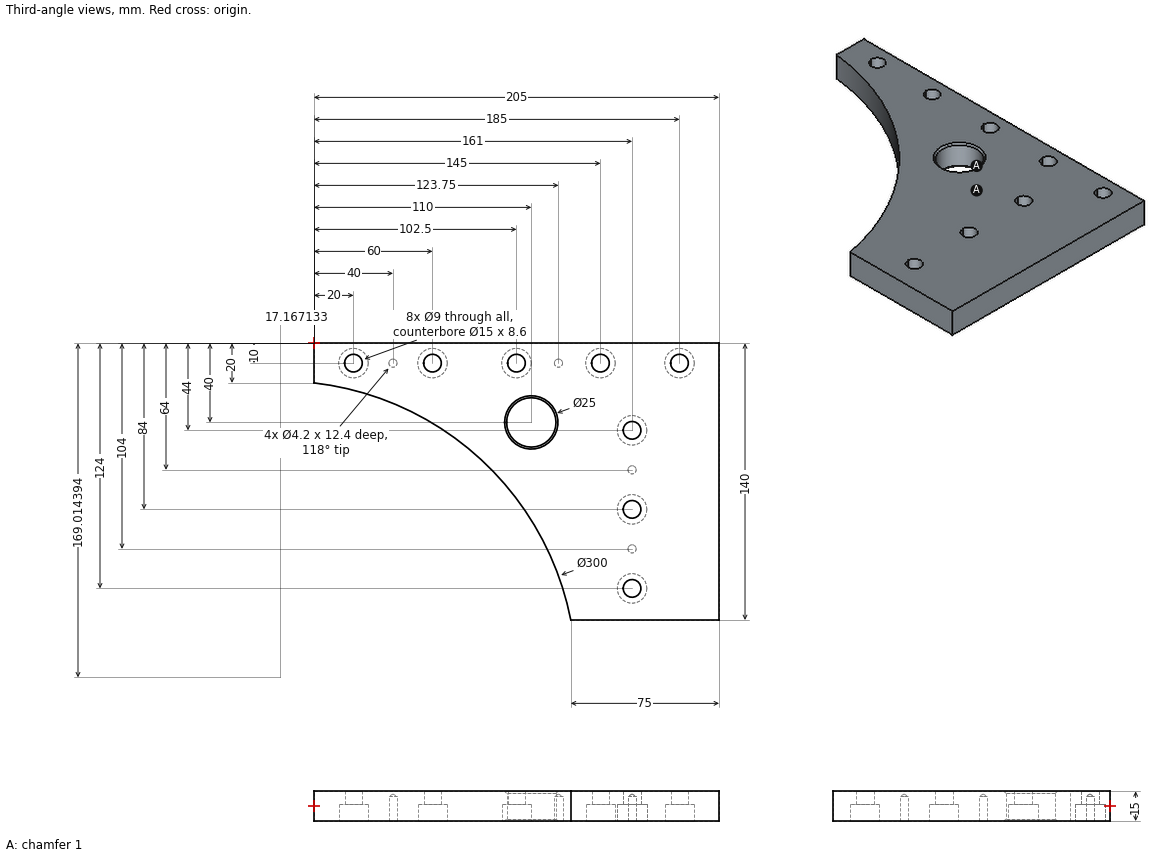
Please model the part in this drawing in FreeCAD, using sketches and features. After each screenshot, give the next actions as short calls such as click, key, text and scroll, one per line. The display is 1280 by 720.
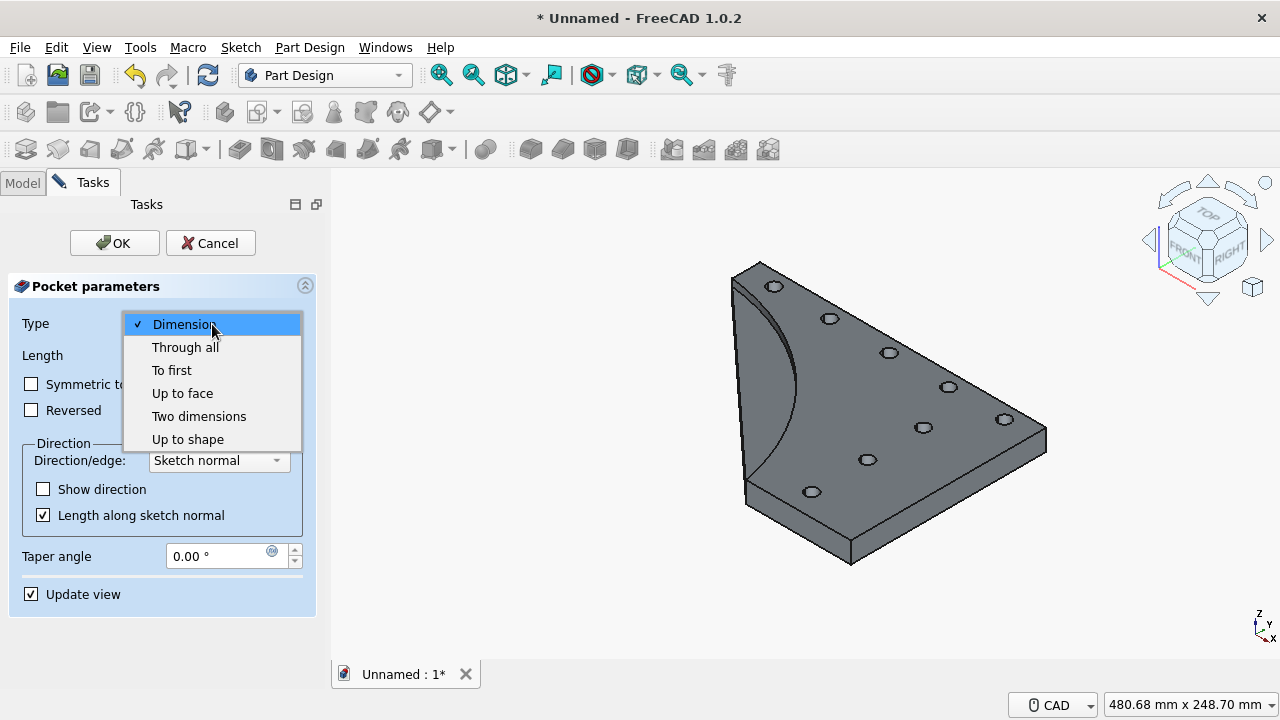
click(212, 348)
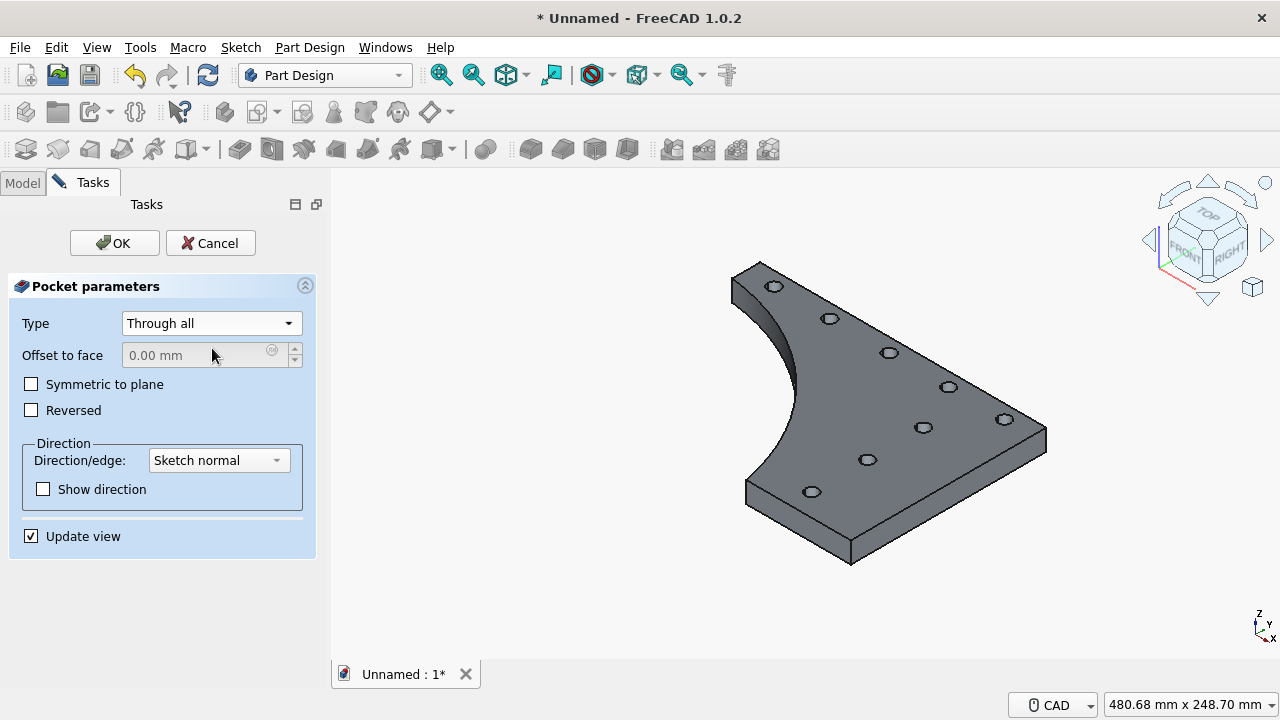
click(115, 243)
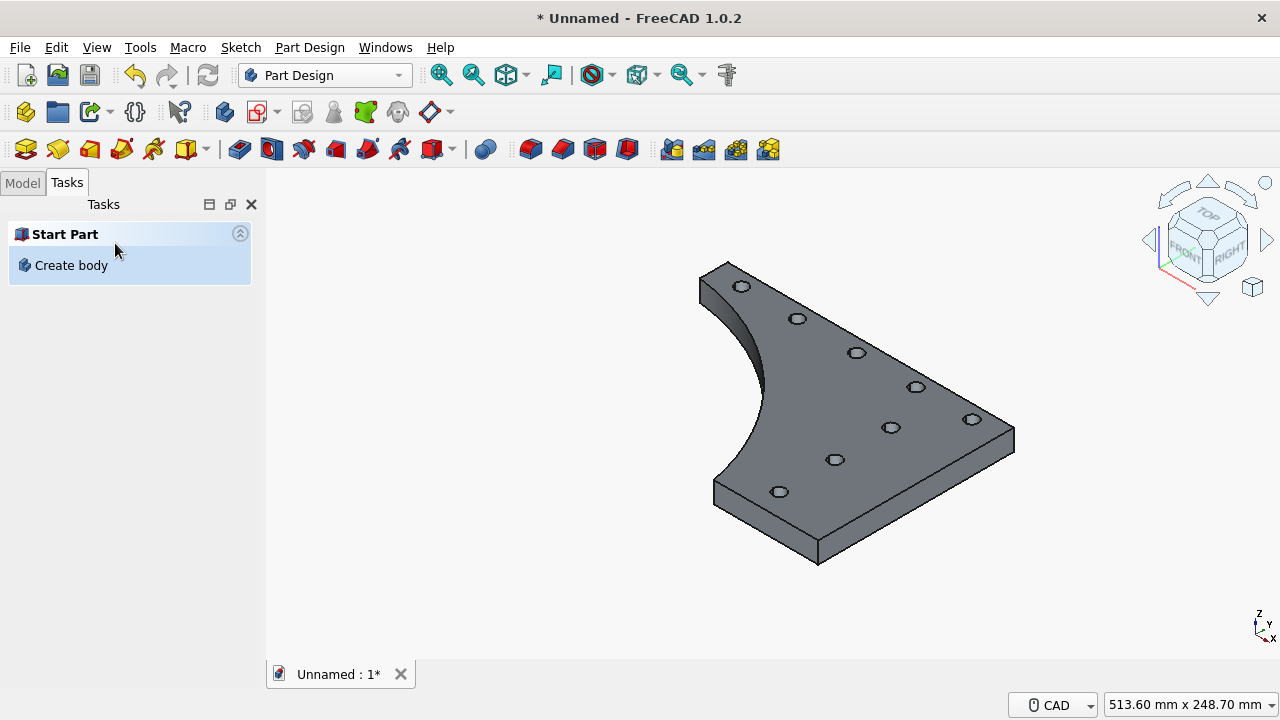
key(5)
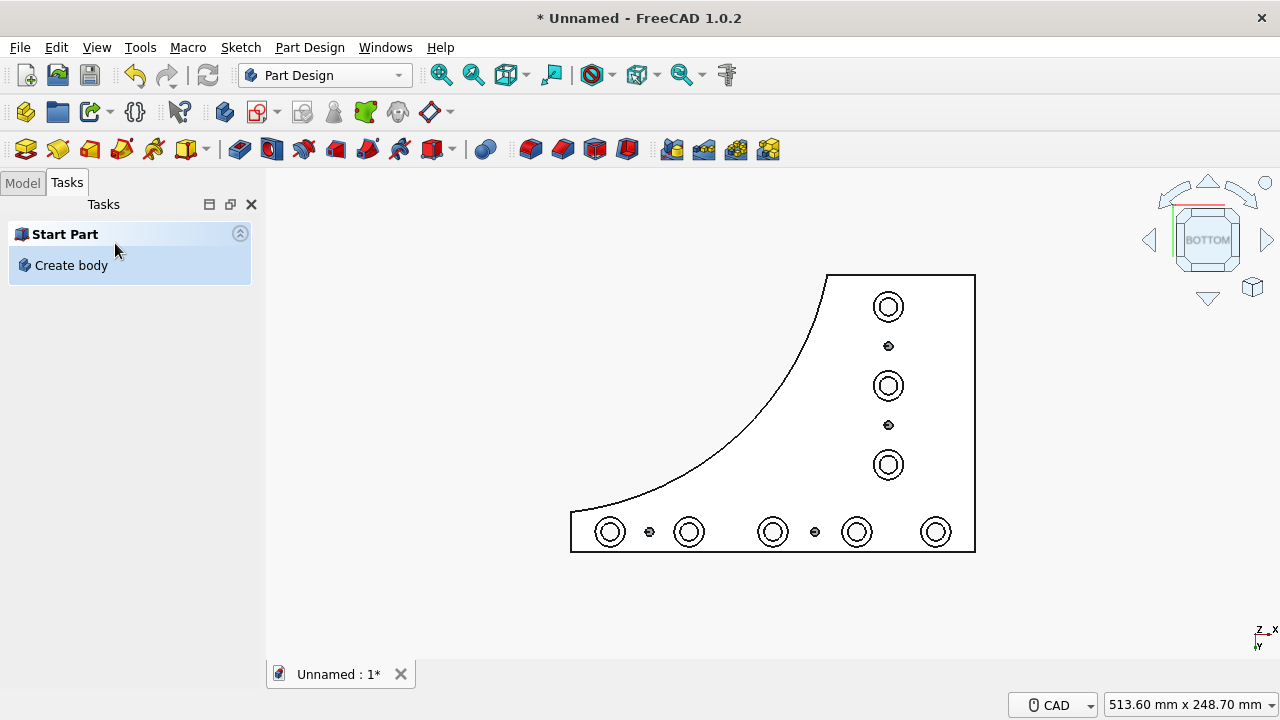
click(831, 413)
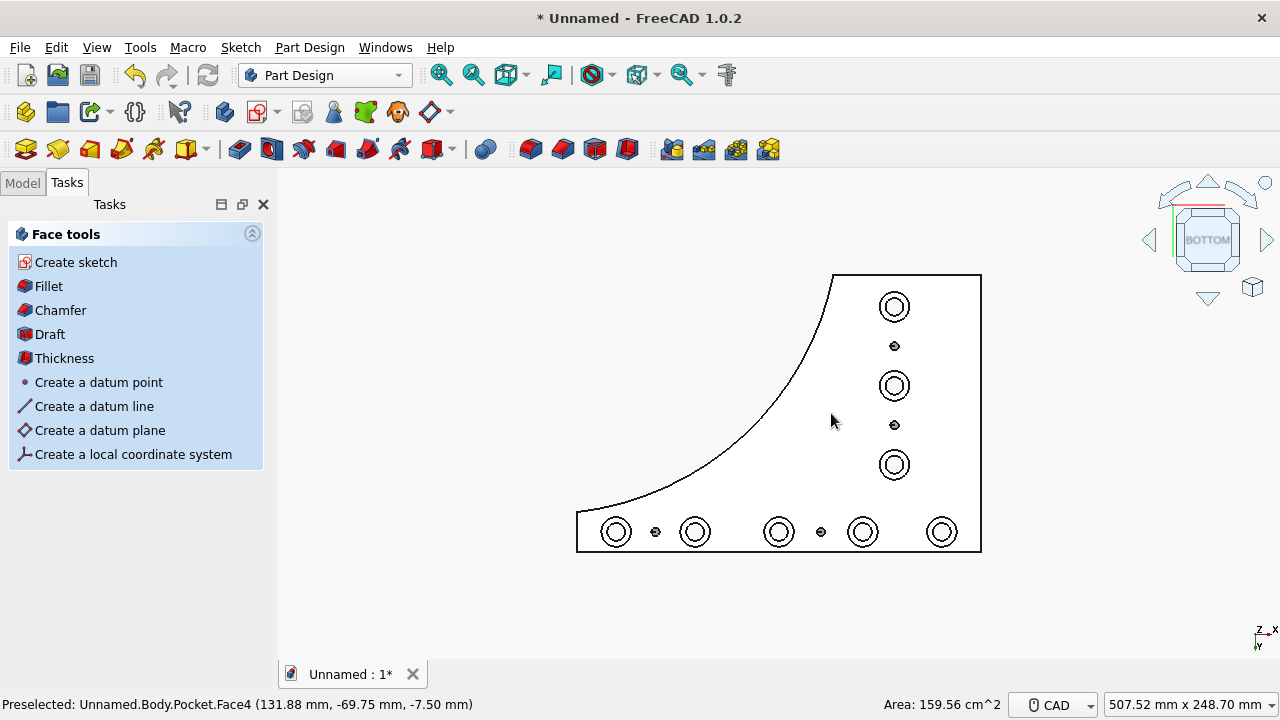
click(258, 112)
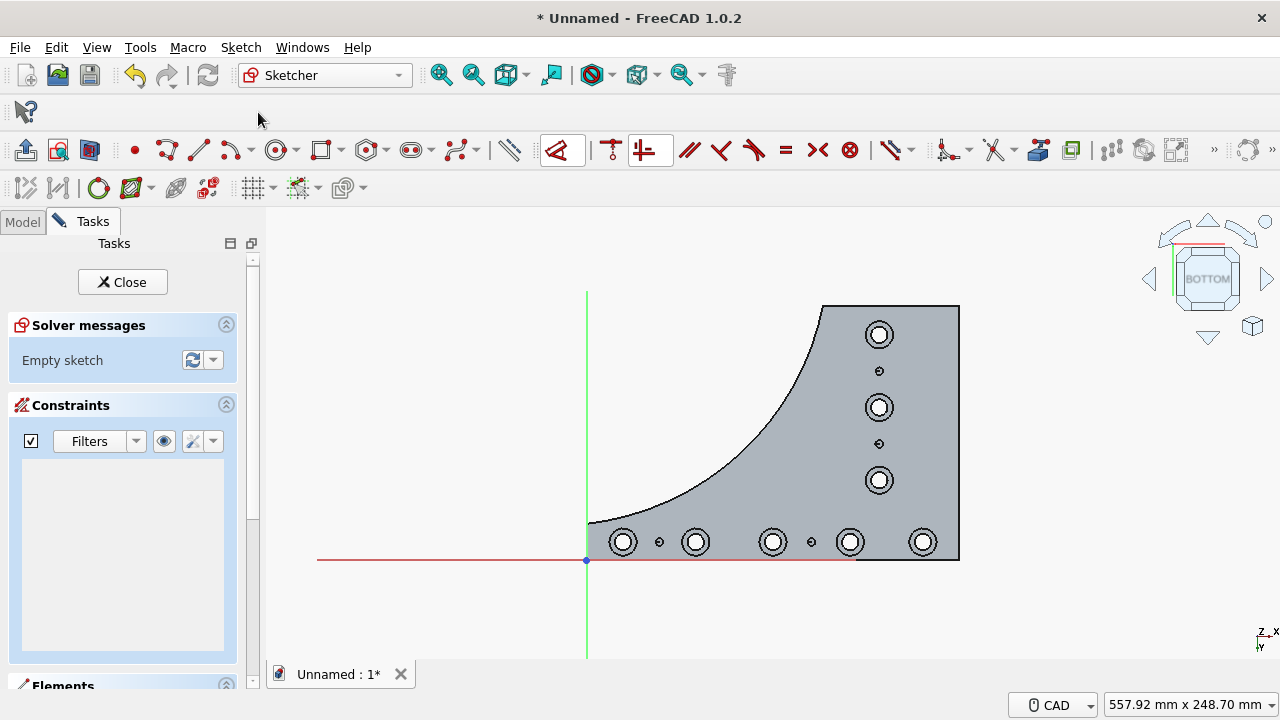
scroll(803, 498, up, 9)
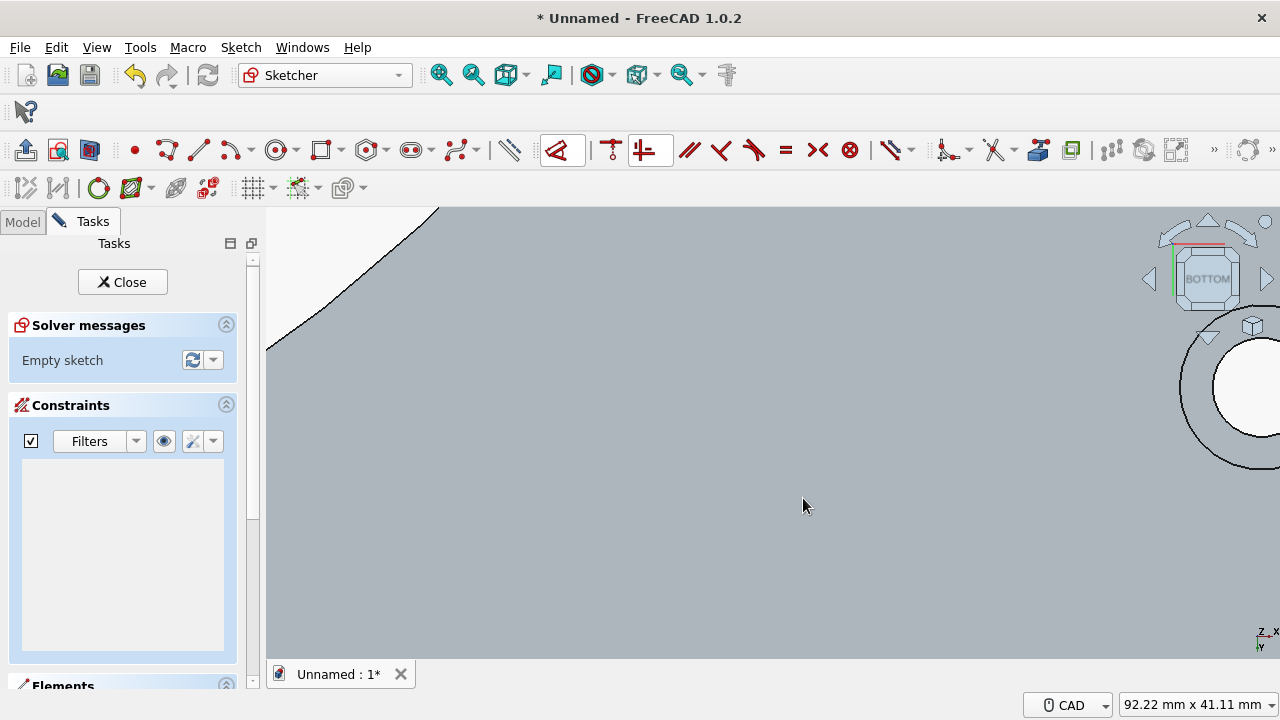
click(276, 150)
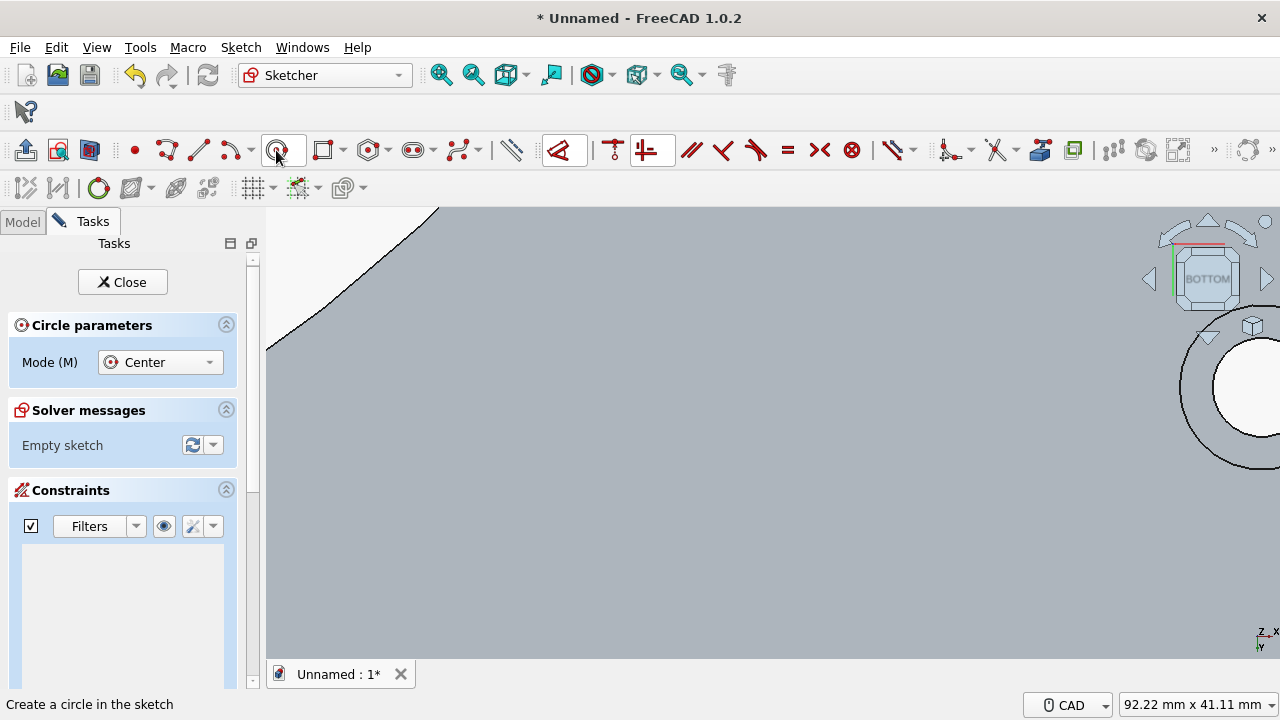
click(701, 431)
click(798, 334)
key(Escape)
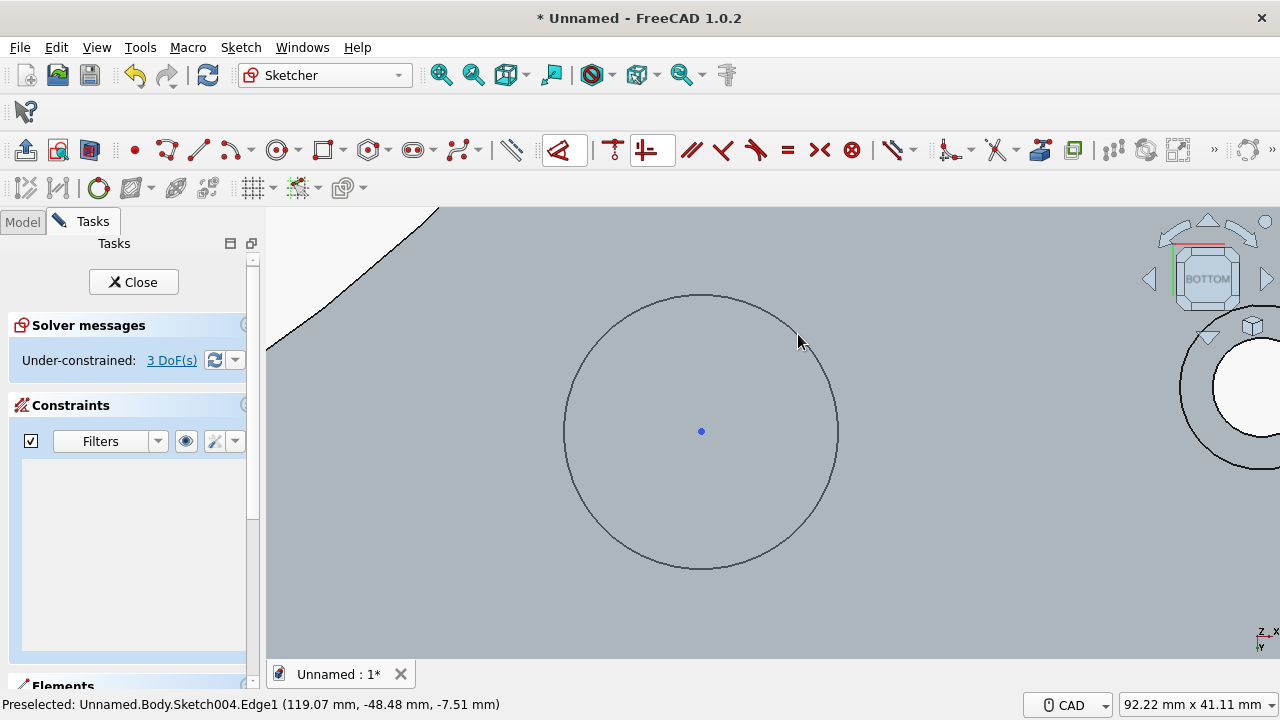
click(798, 335)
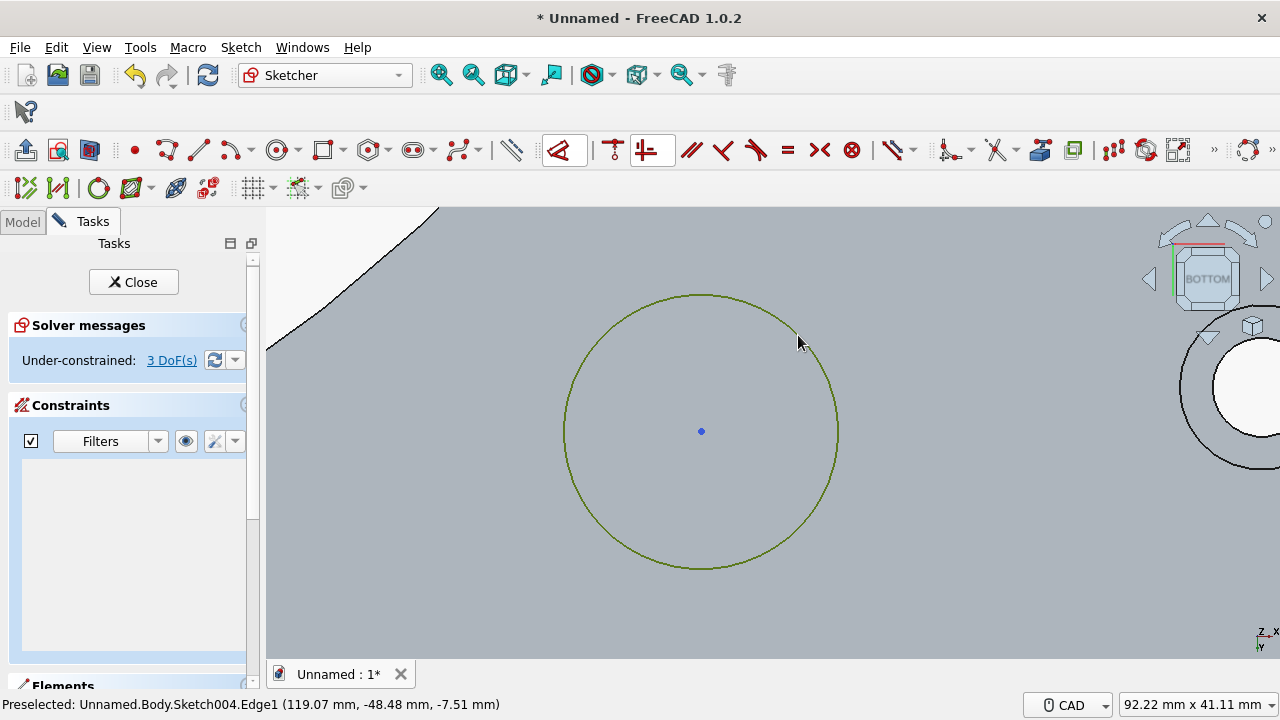
click(582, 150)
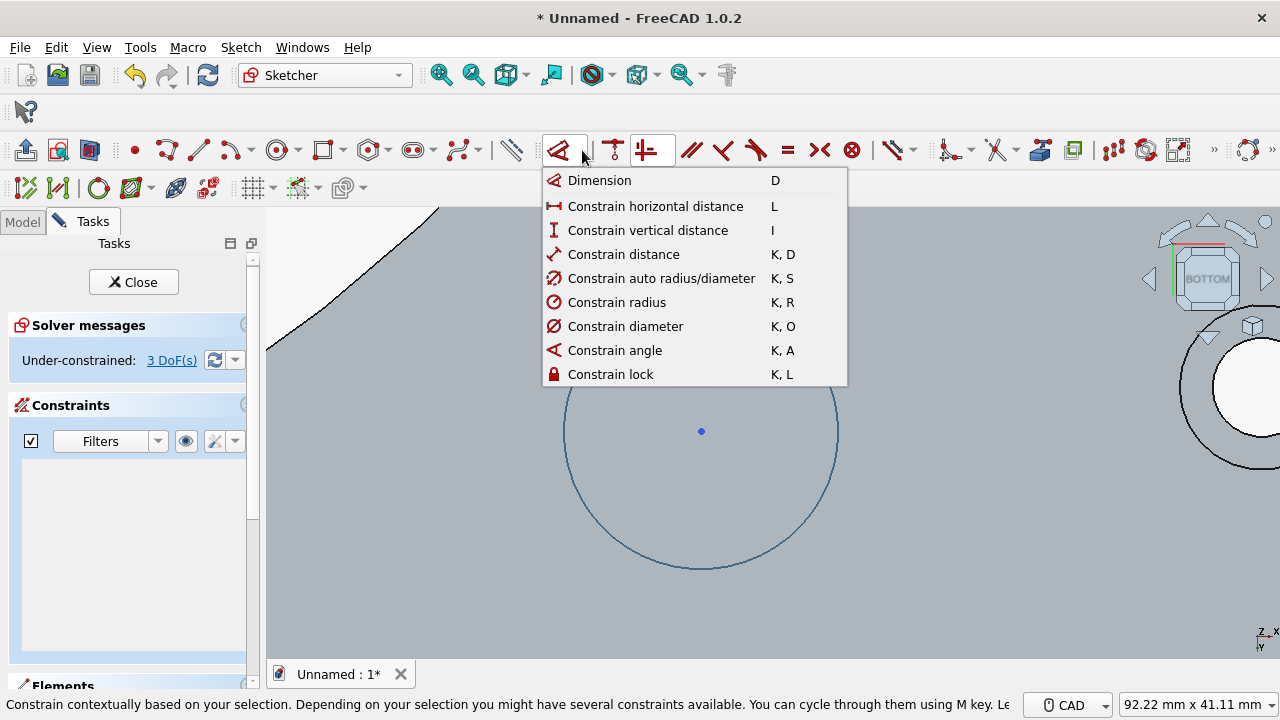
click(695, 326)